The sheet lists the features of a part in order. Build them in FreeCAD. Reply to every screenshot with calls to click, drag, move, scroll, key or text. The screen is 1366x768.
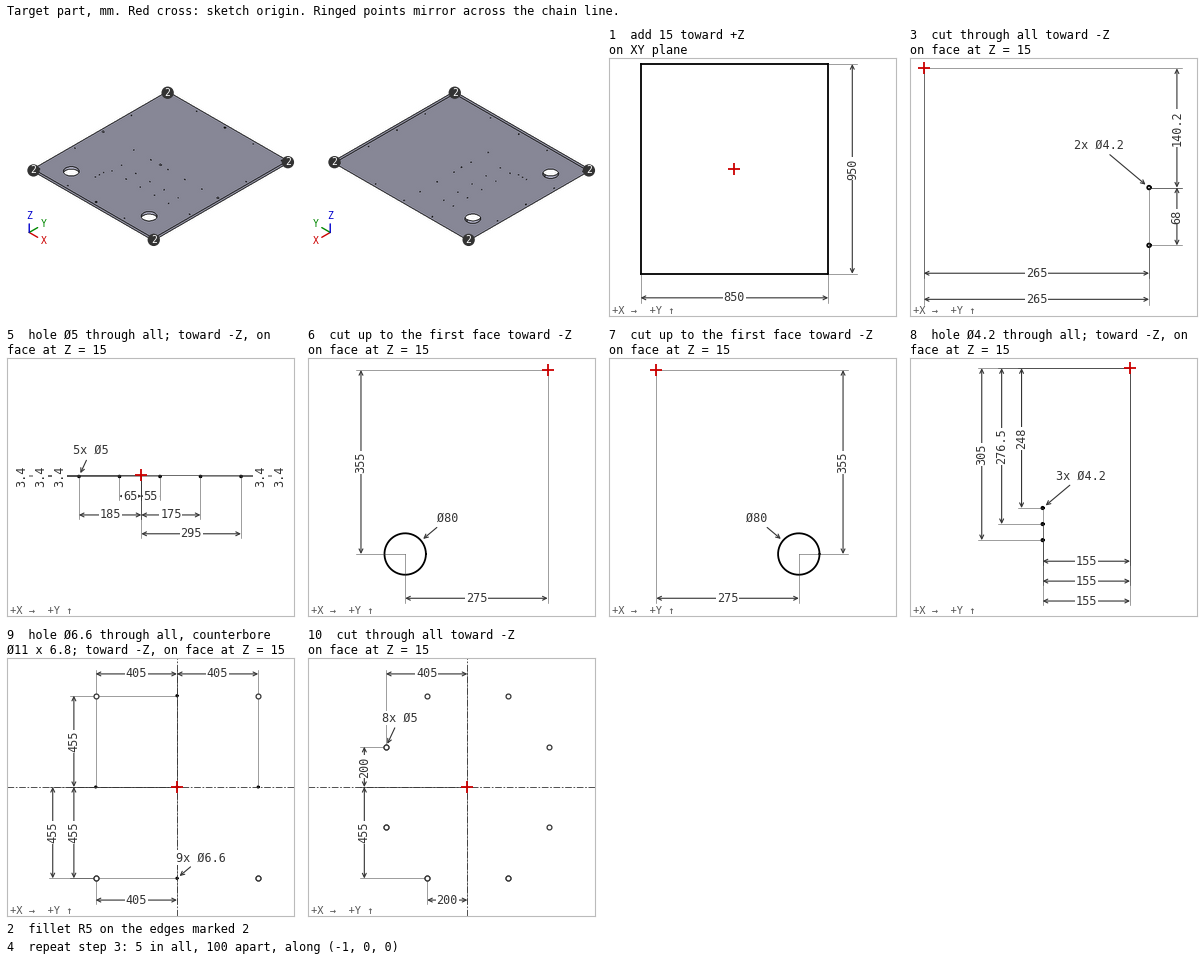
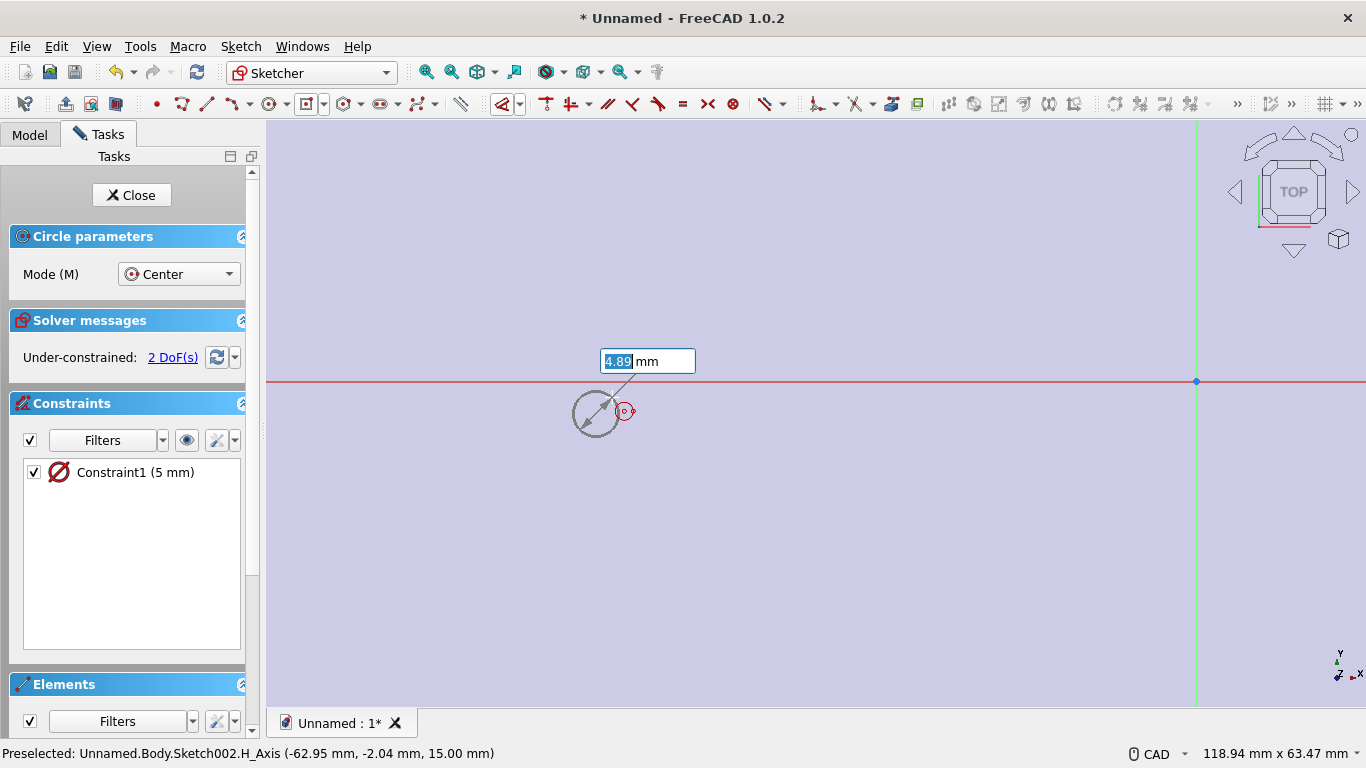
text(5)
key(Return)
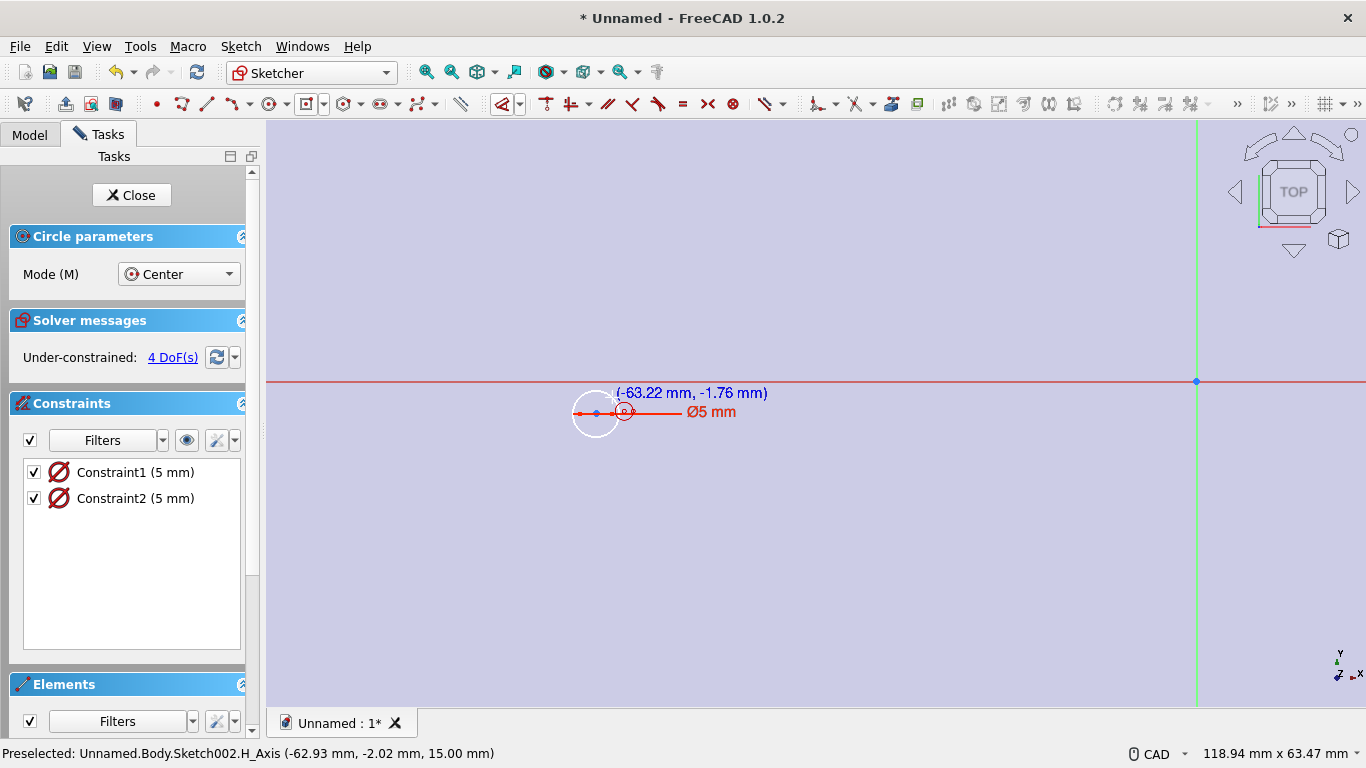
scroll(598, 414, down, 10)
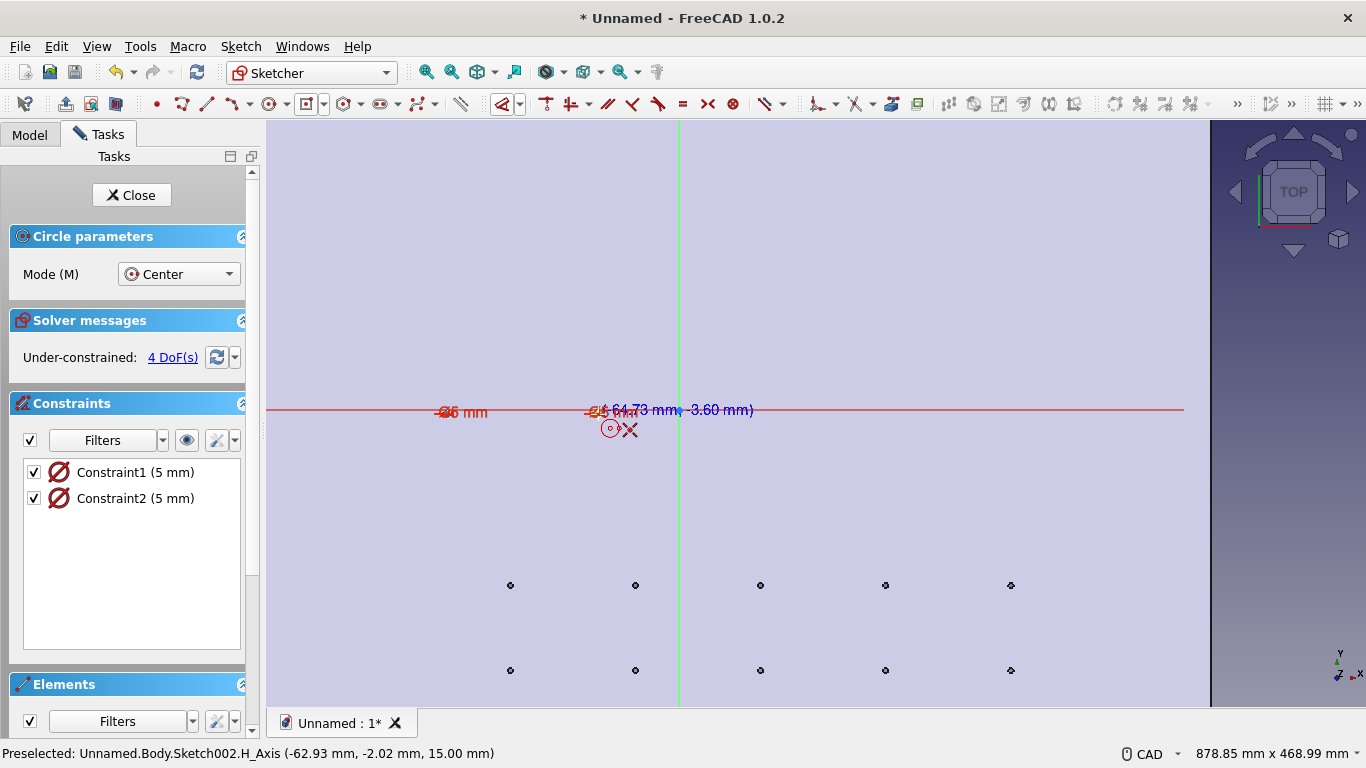
scroll(748, 414, up, 10)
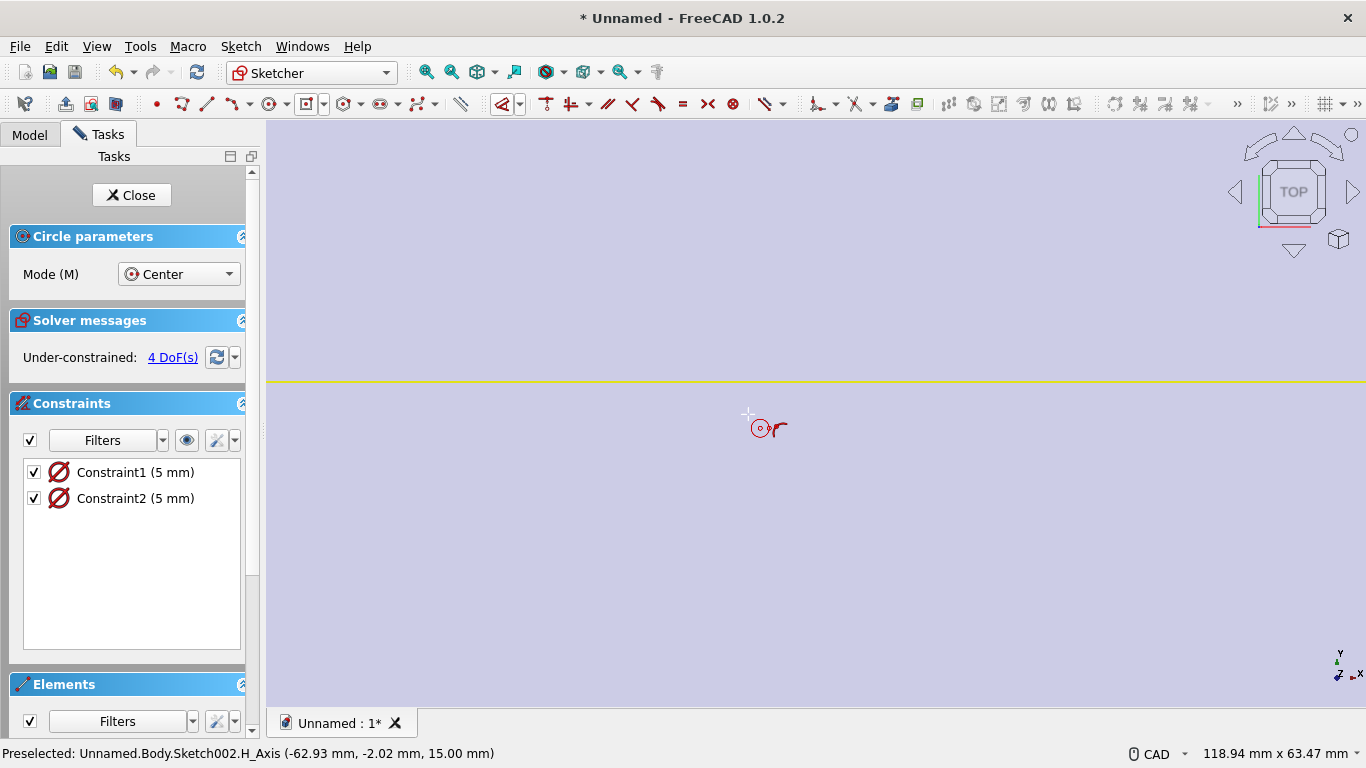
click(746, 413)
move(762, 397)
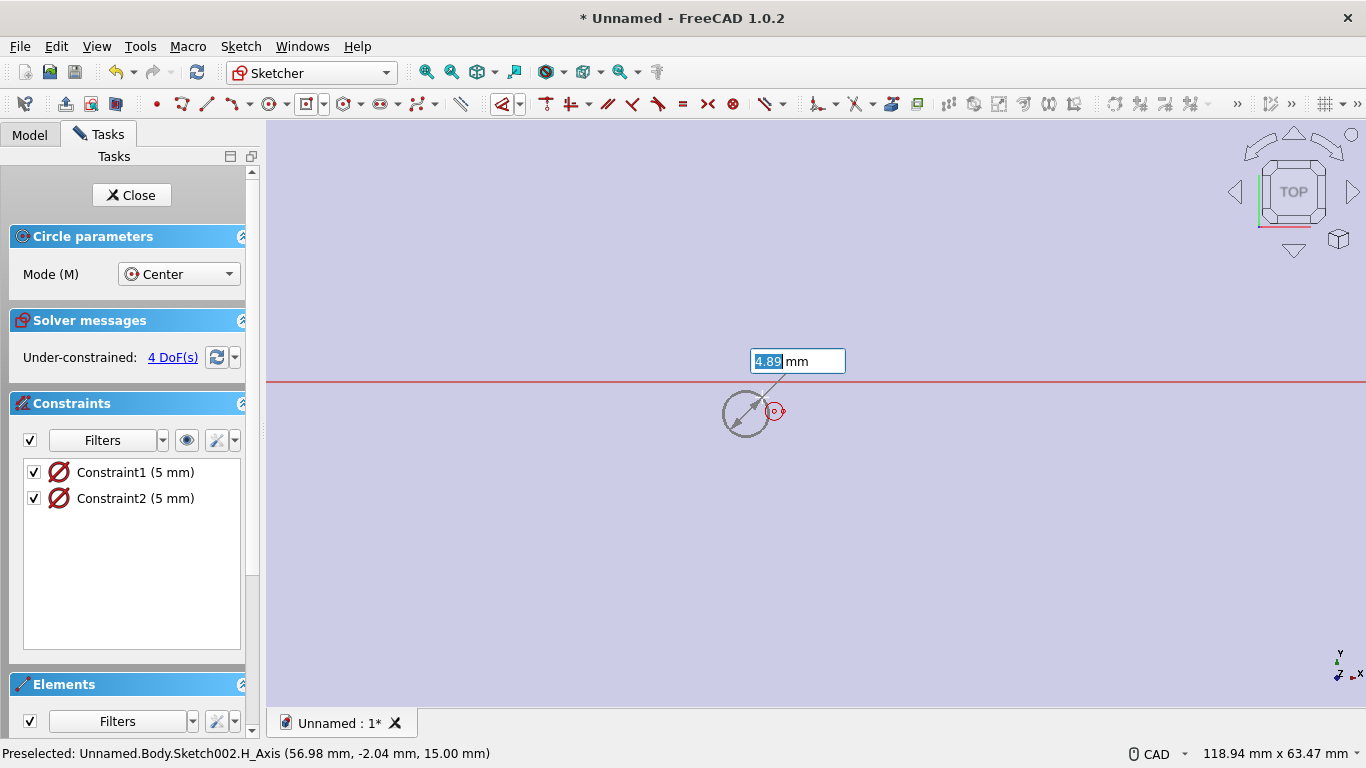
text(5)
key(Return)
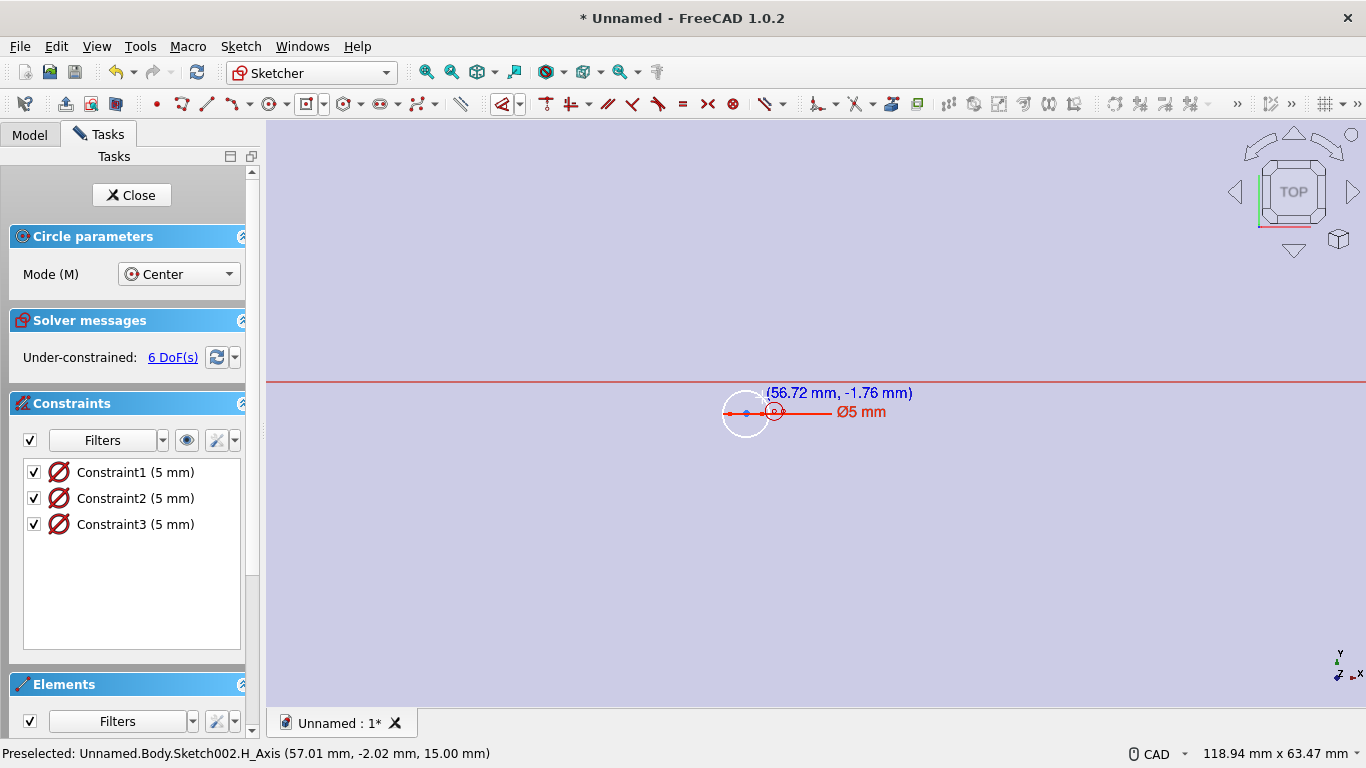
scroll(748, 414, down, 10)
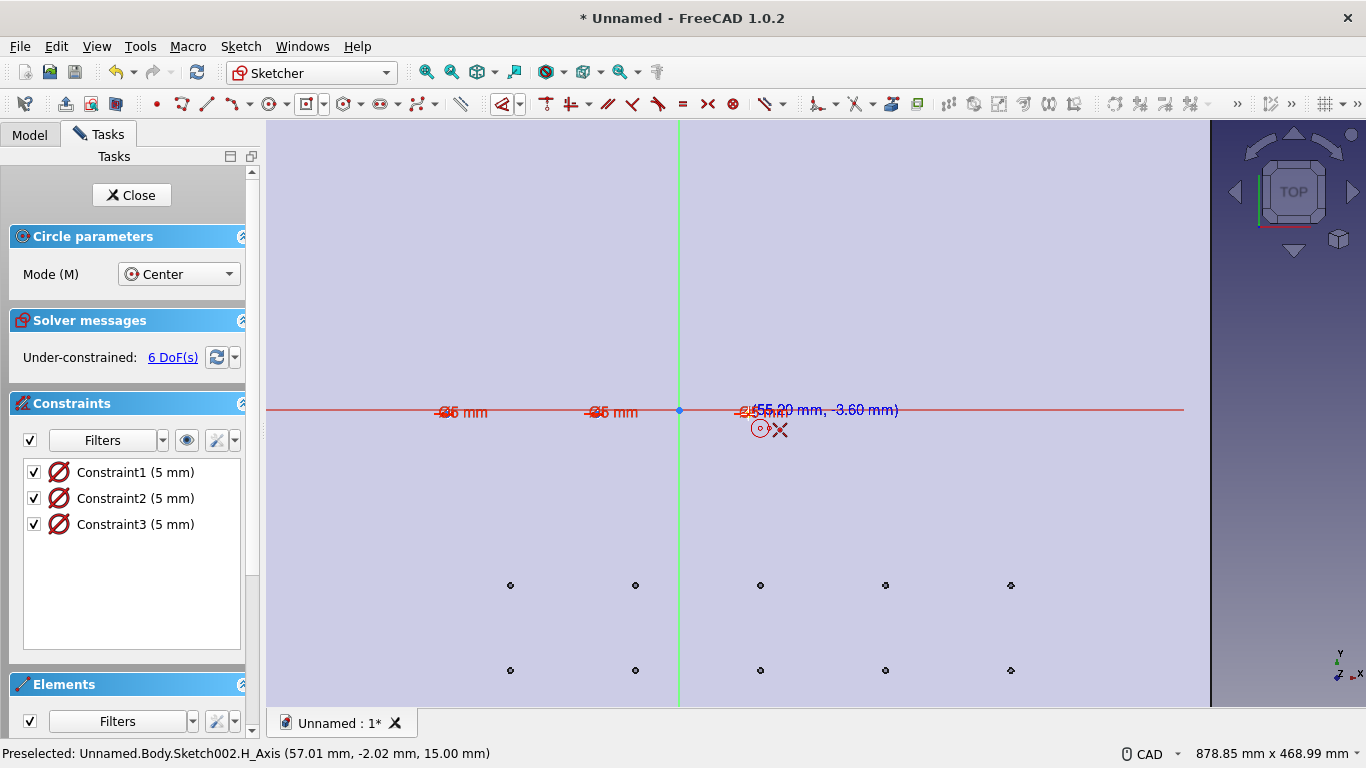
scroll(898, 414, up, 10)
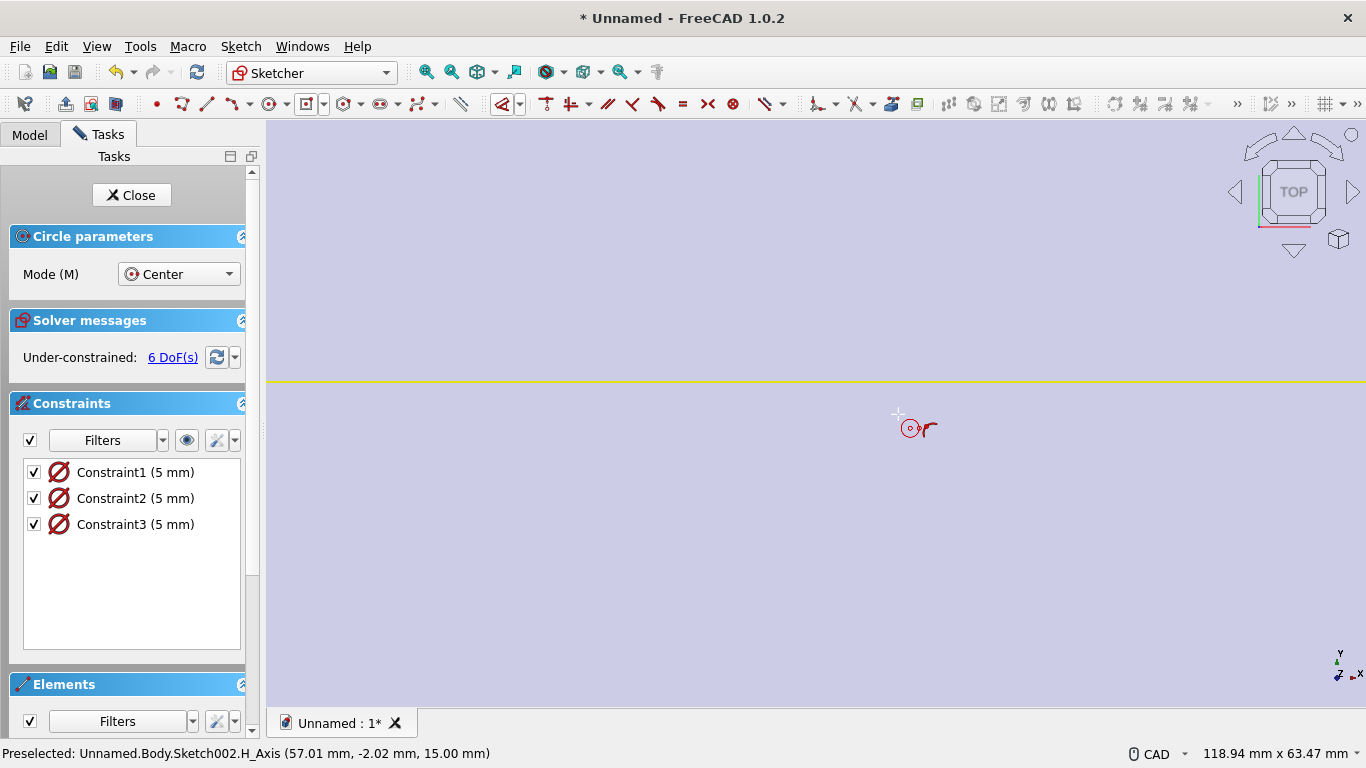
click(897, 413)
move(913, 397)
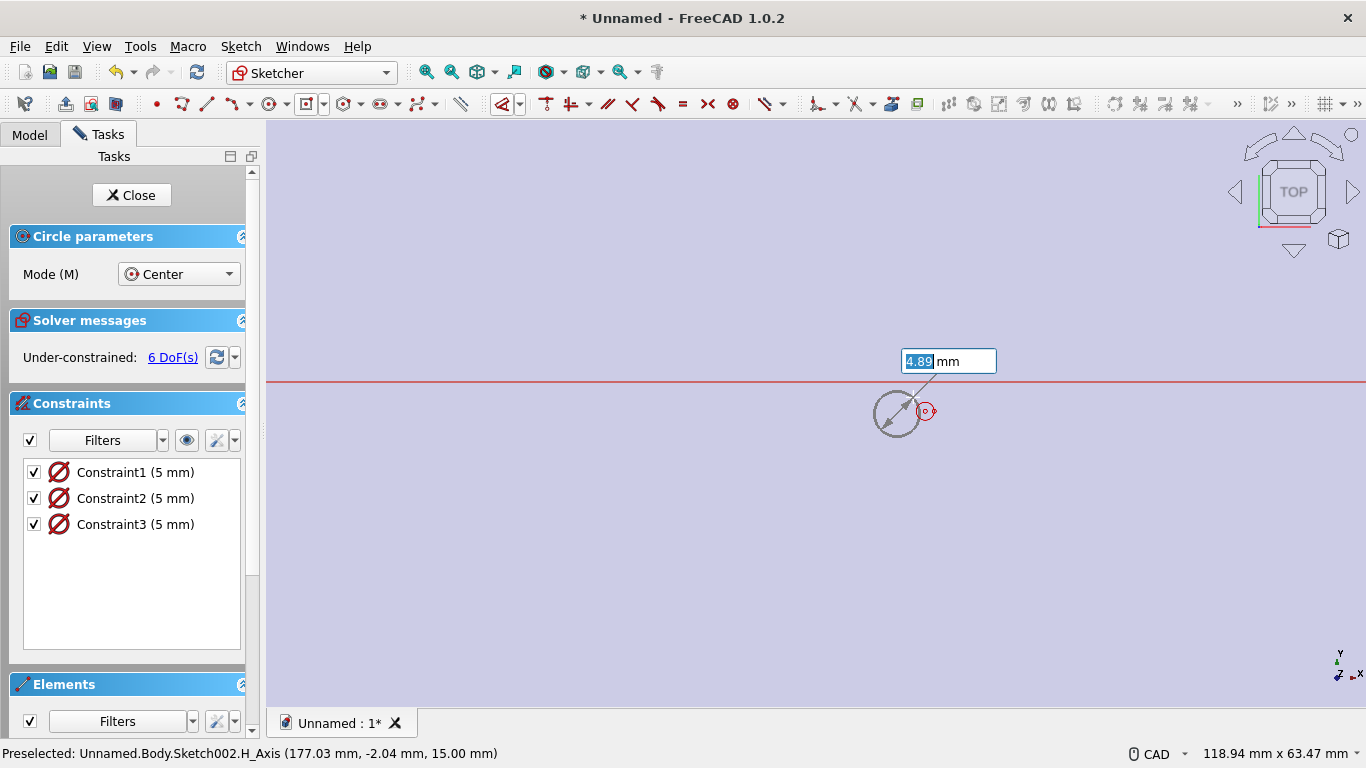
text(5)
key(Return)